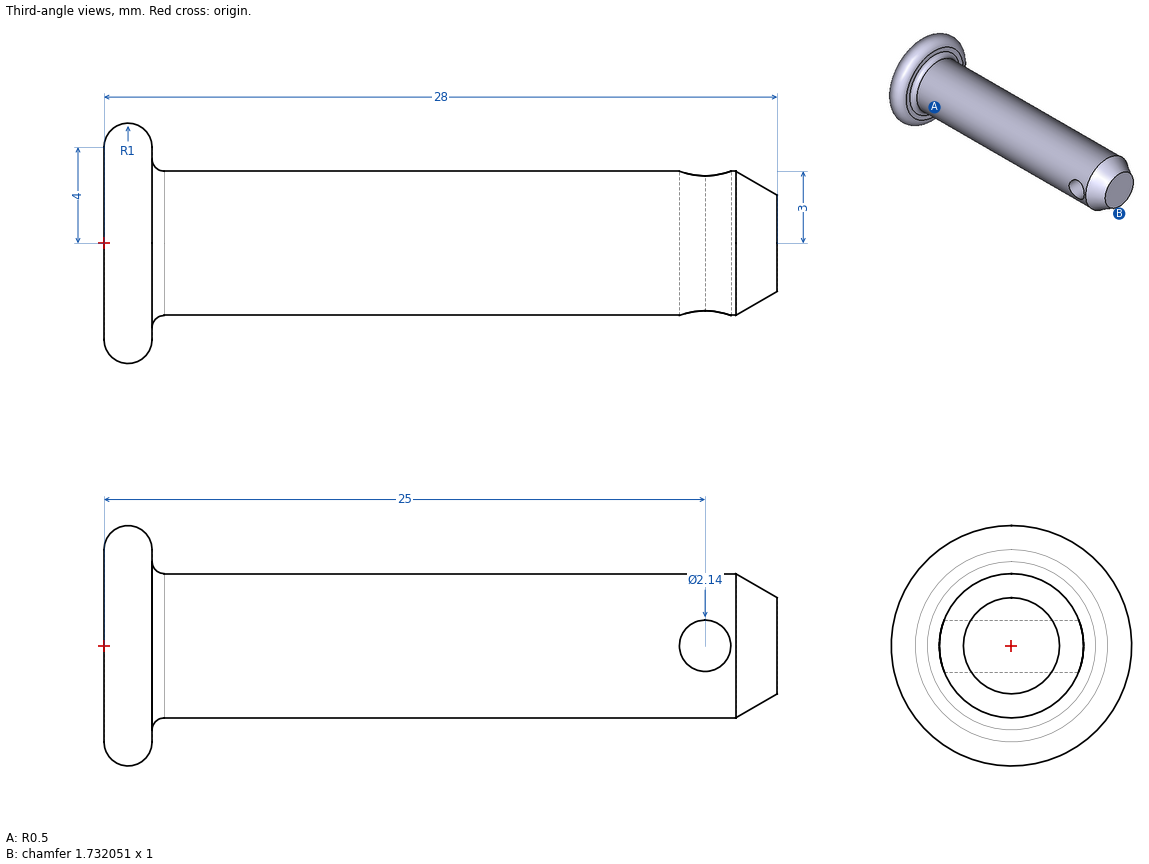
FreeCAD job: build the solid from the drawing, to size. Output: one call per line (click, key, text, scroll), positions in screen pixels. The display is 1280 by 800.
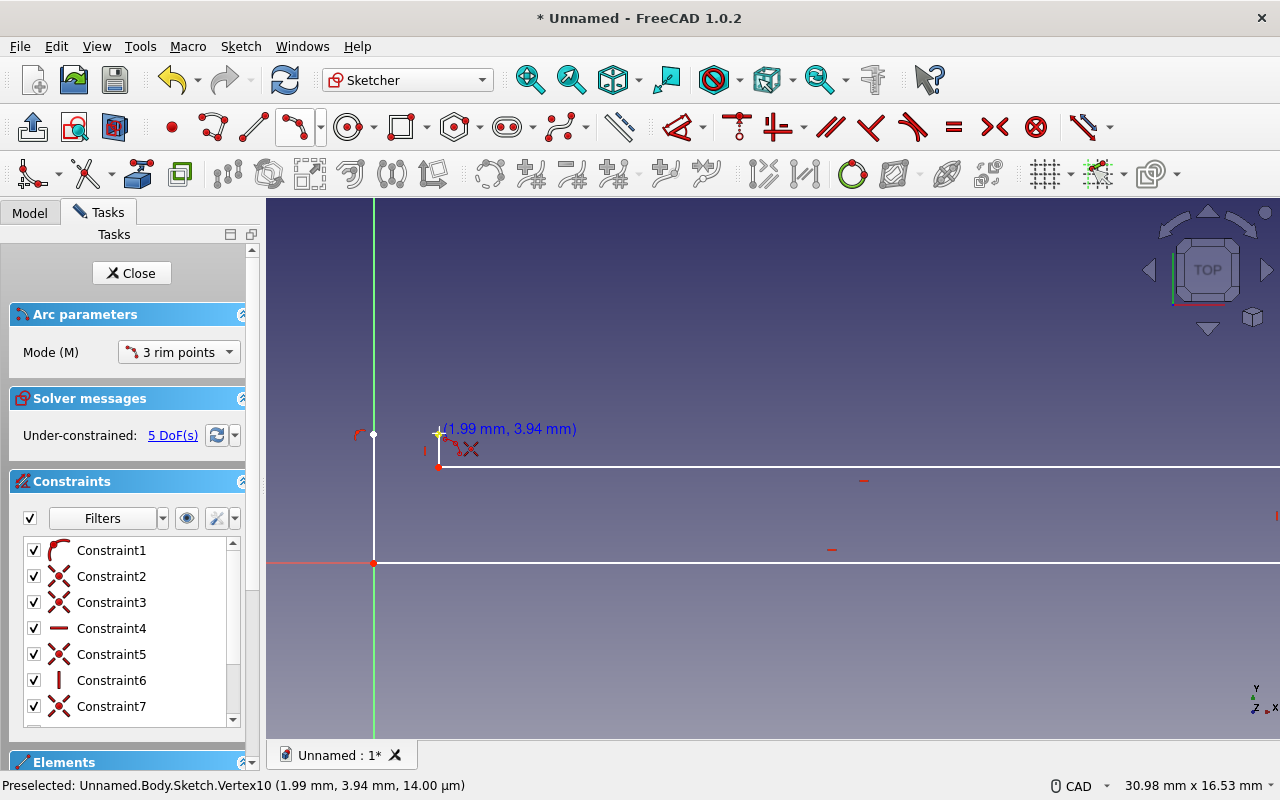
click(439, 434)
click(374, 434)
click(406, 400)
key(Escape)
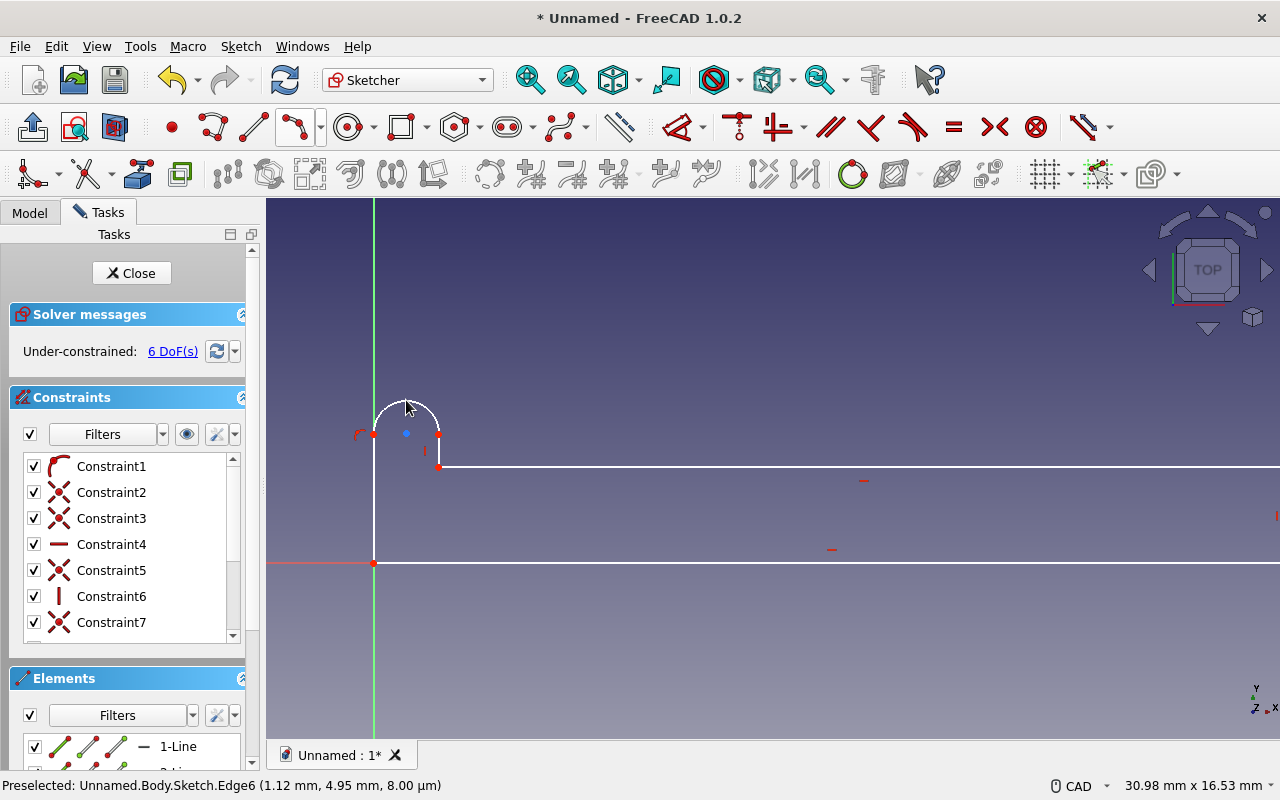
click(374, 473)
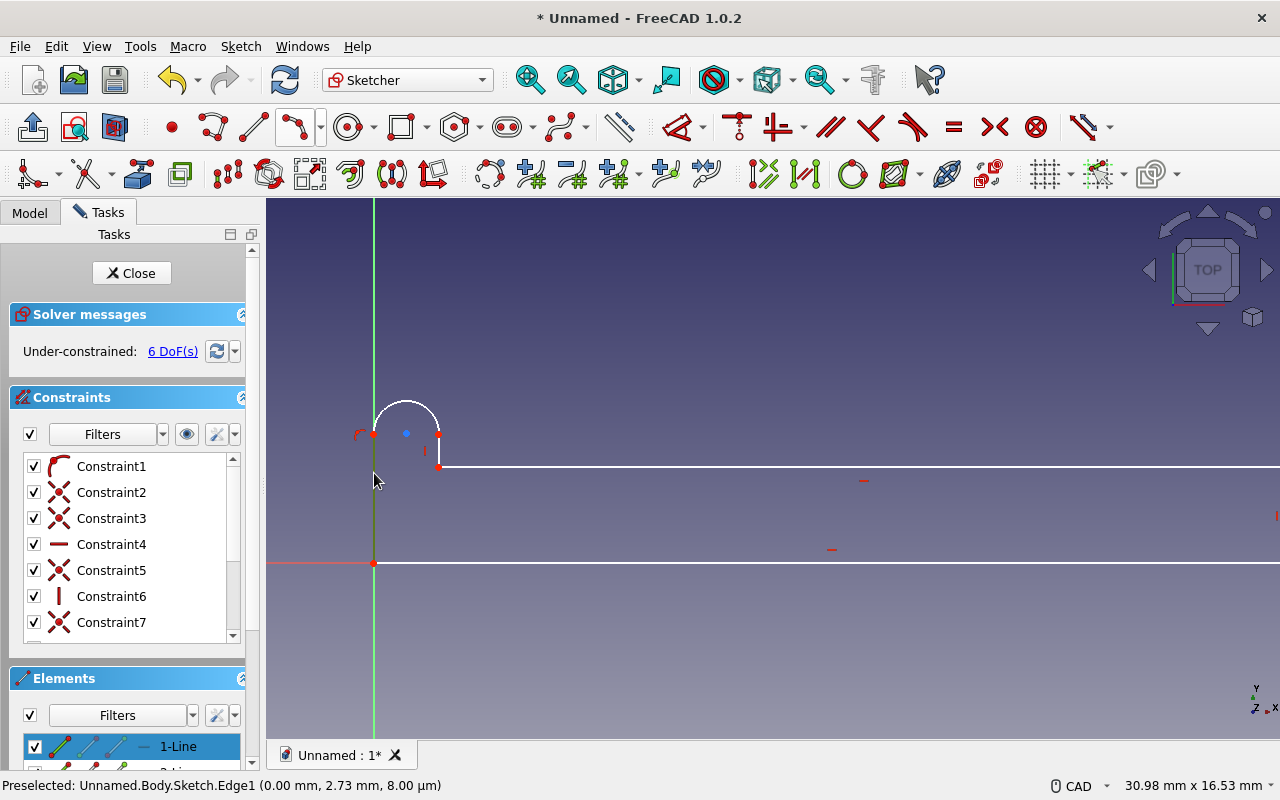
click(426, 407)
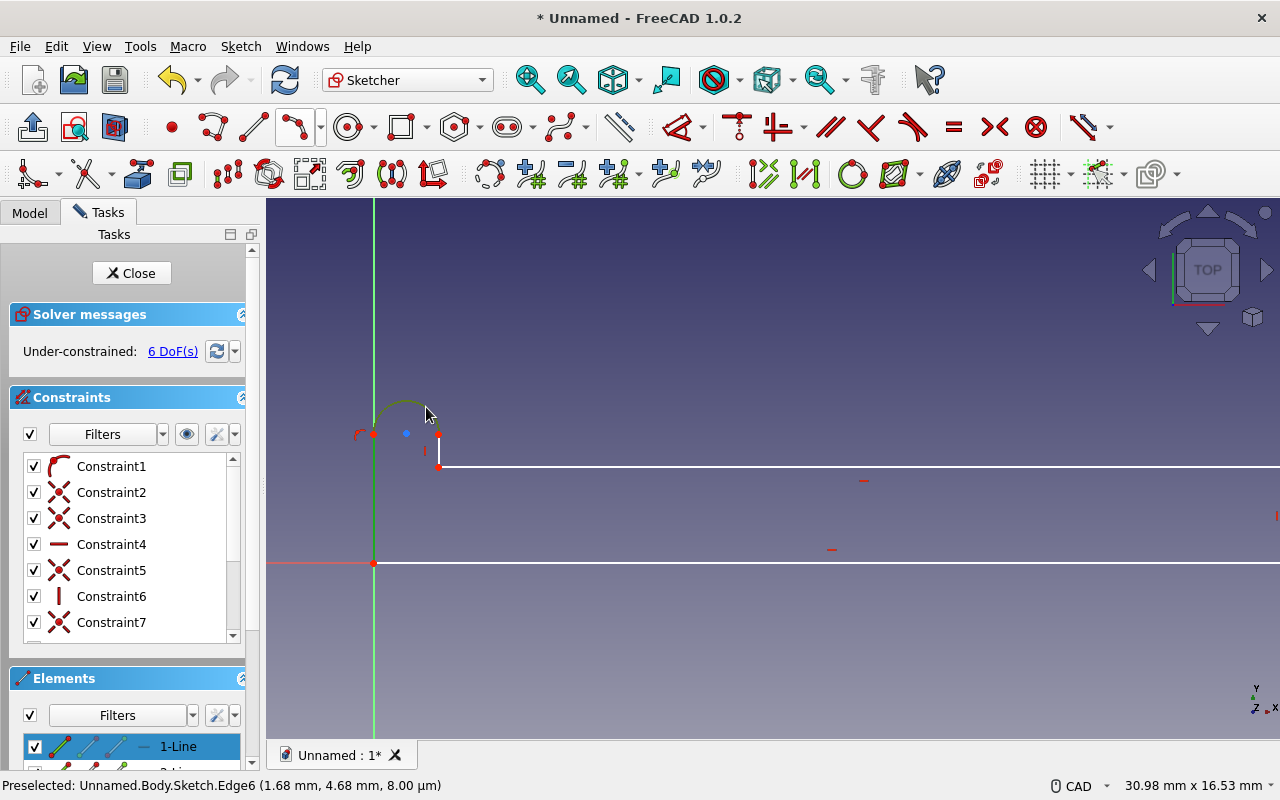
key(t)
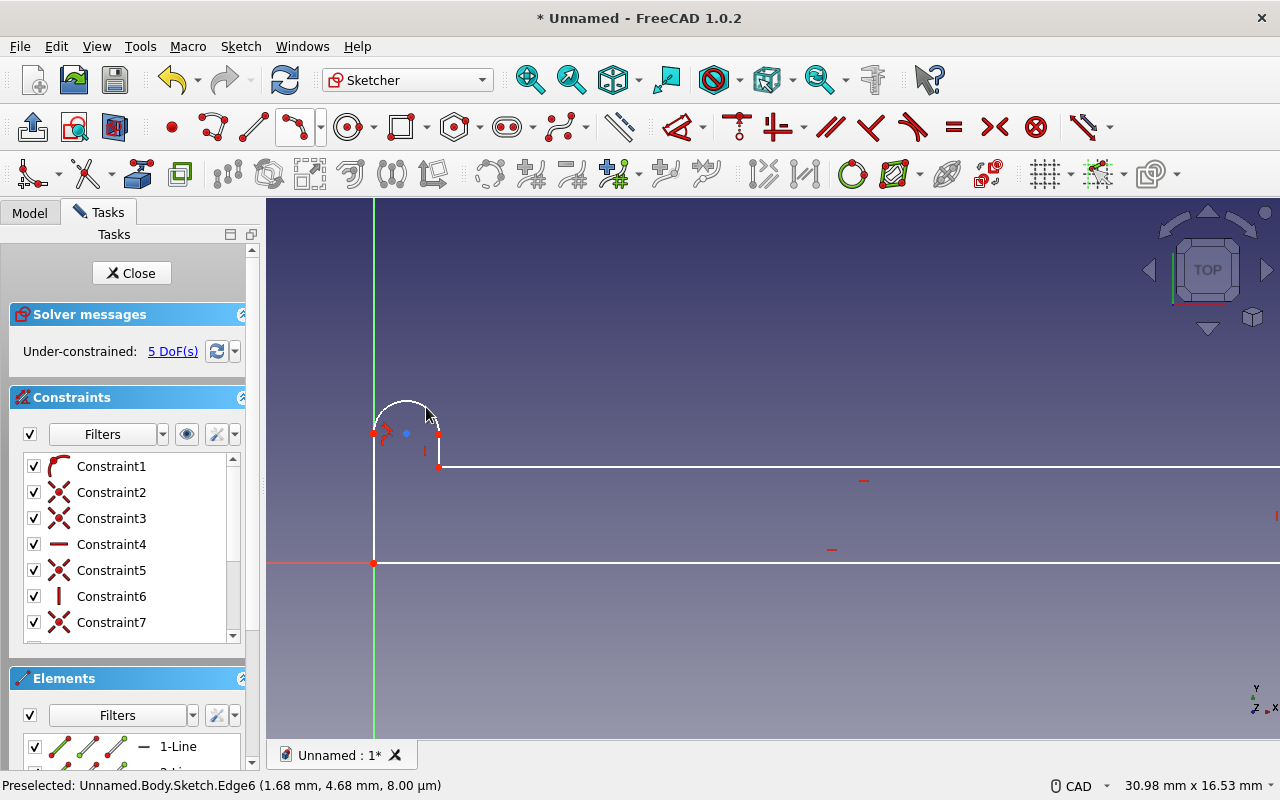
scroll(439, 457, up, 2)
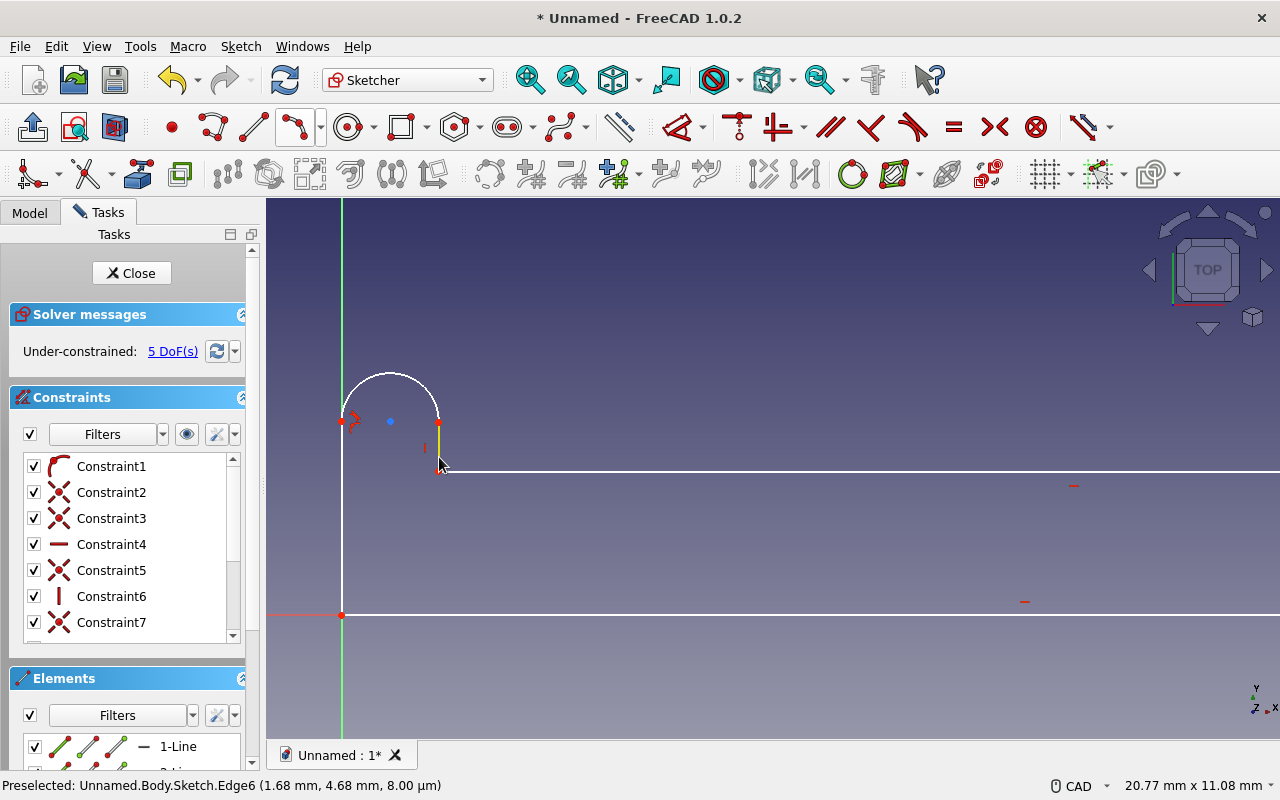
click(439, 457)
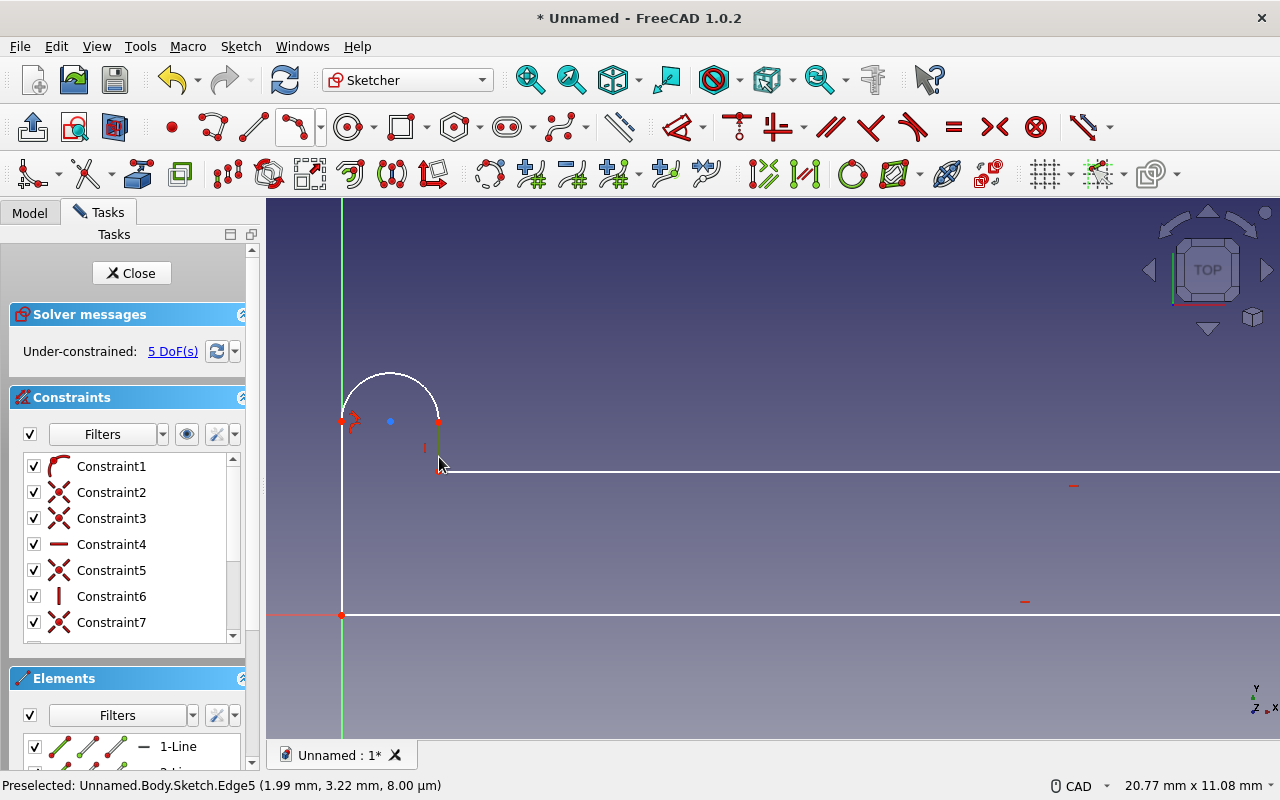
click(419, 383)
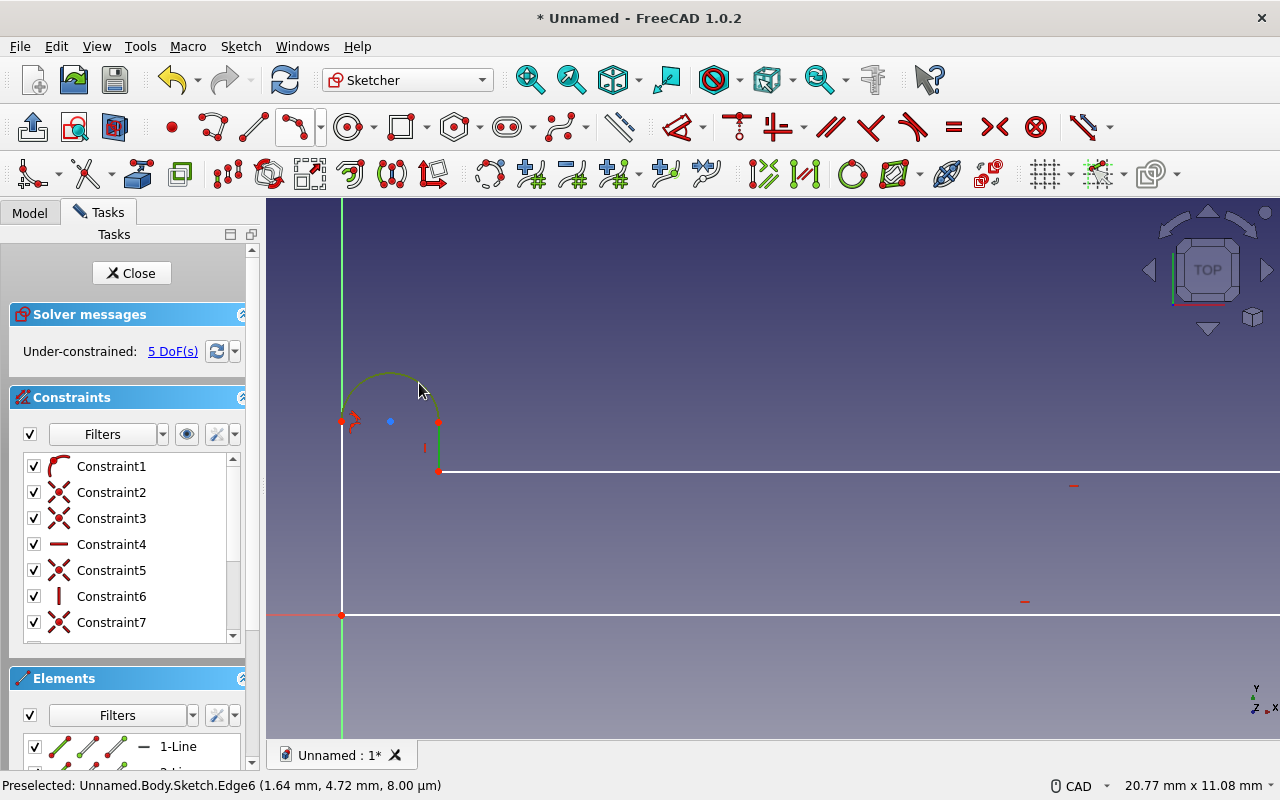
click(913, 128)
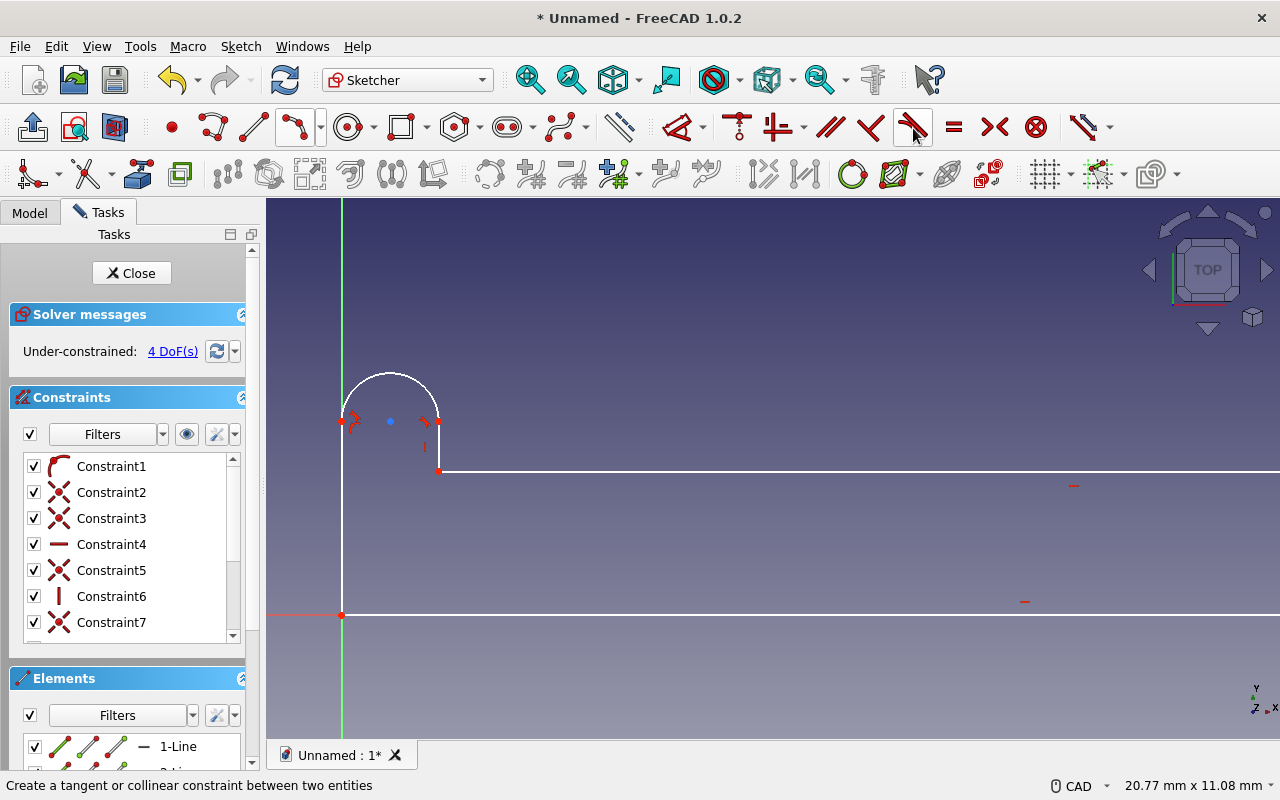
click(419, 383)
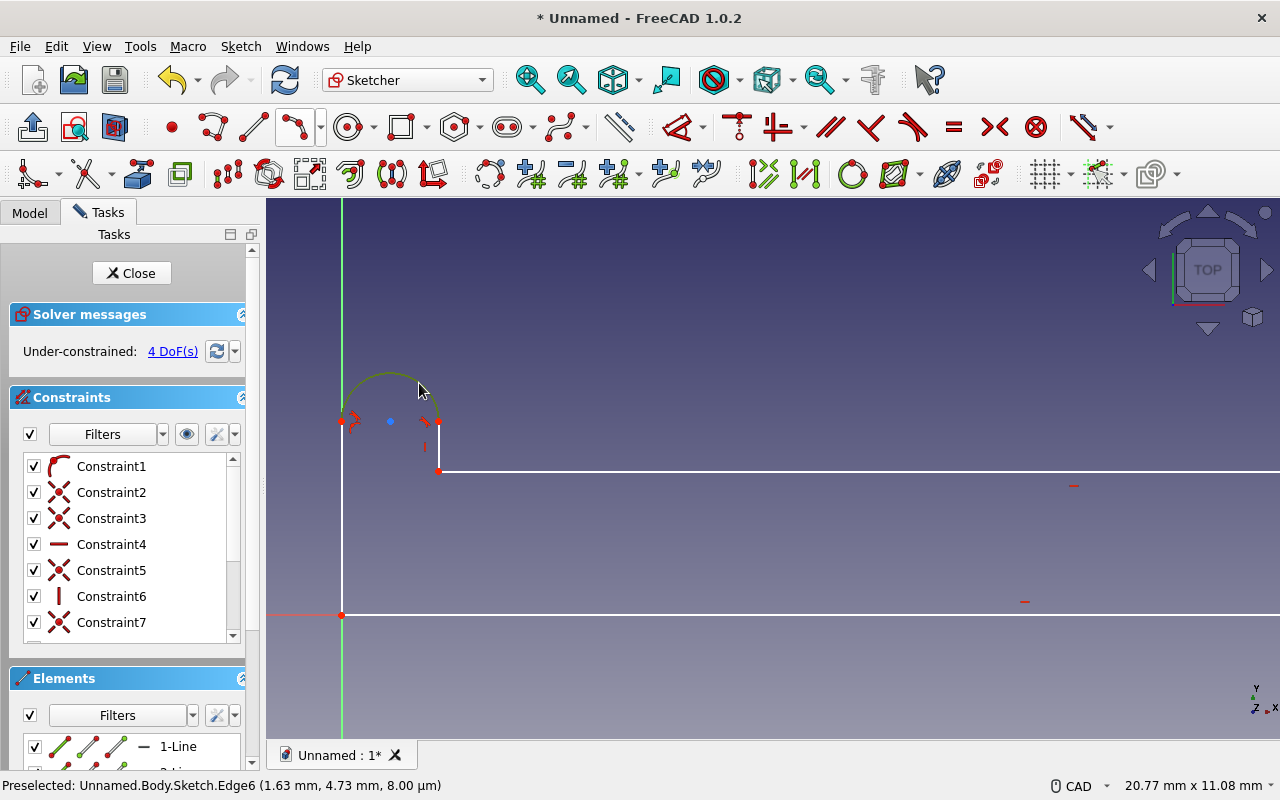
key(k)
key(r)